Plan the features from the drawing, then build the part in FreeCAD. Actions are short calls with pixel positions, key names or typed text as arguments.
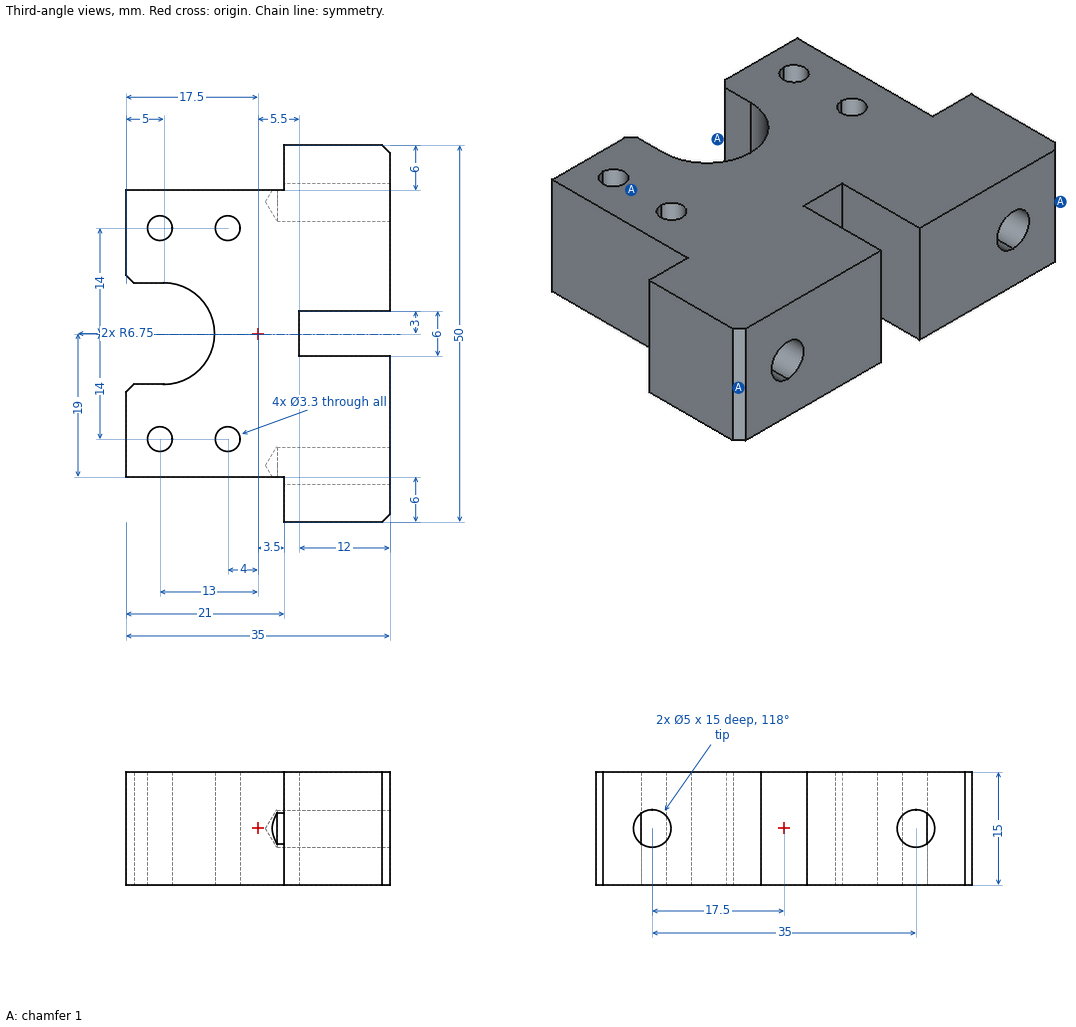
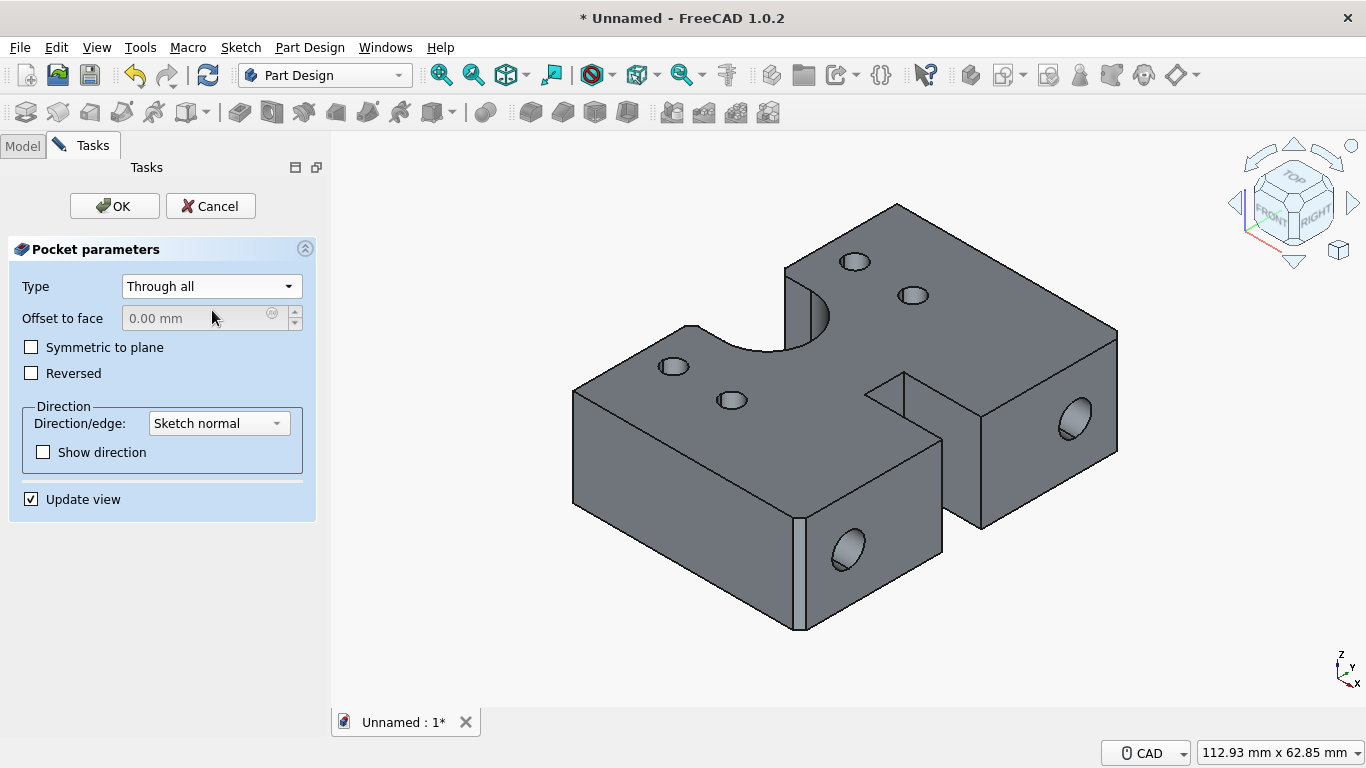
click(115, 206)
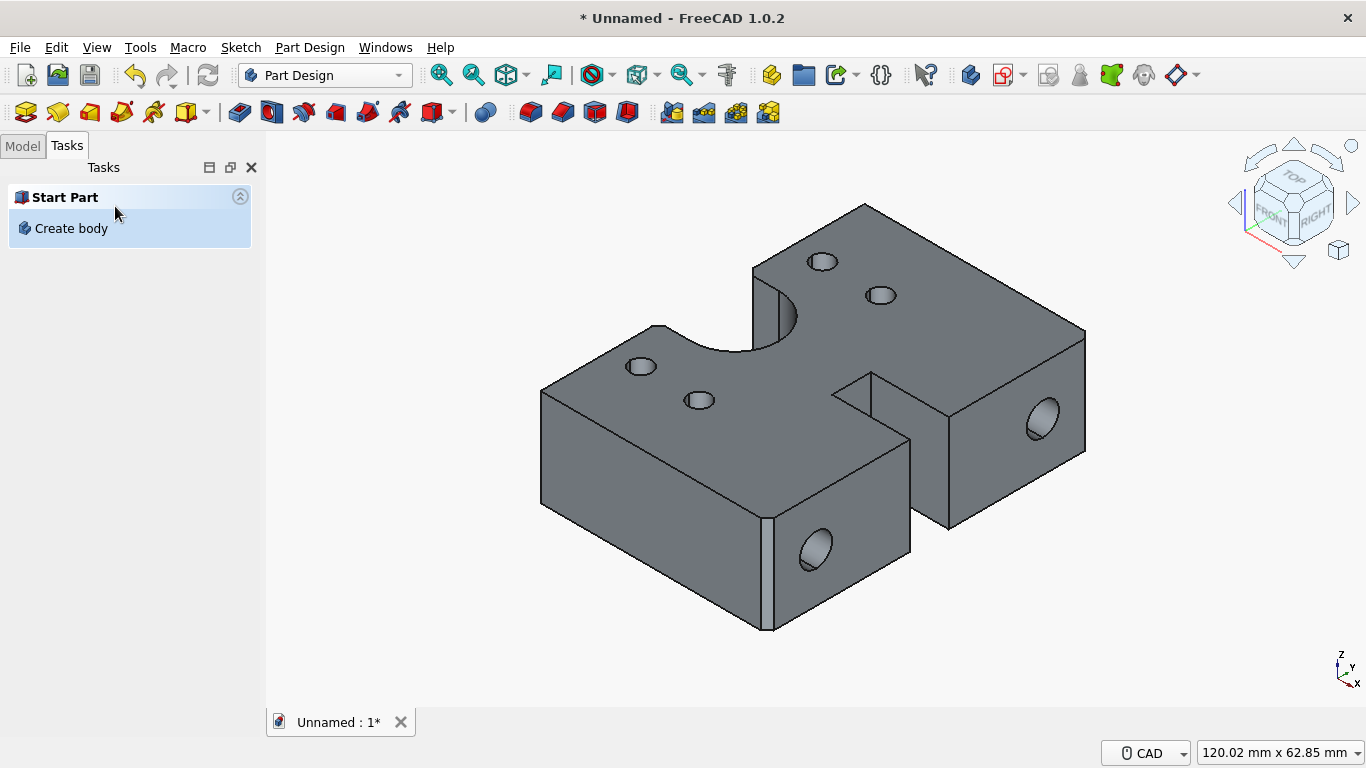
click(973, 346)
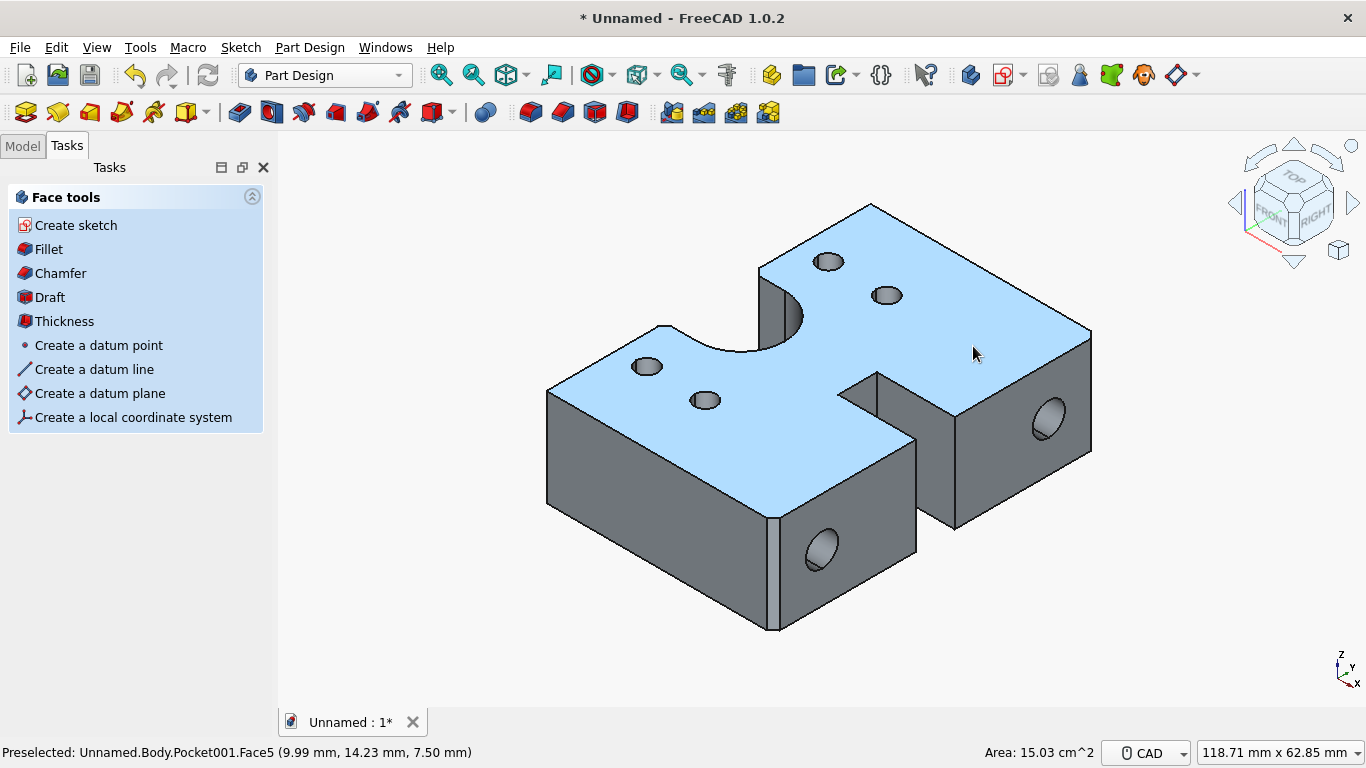
click(1004, 76)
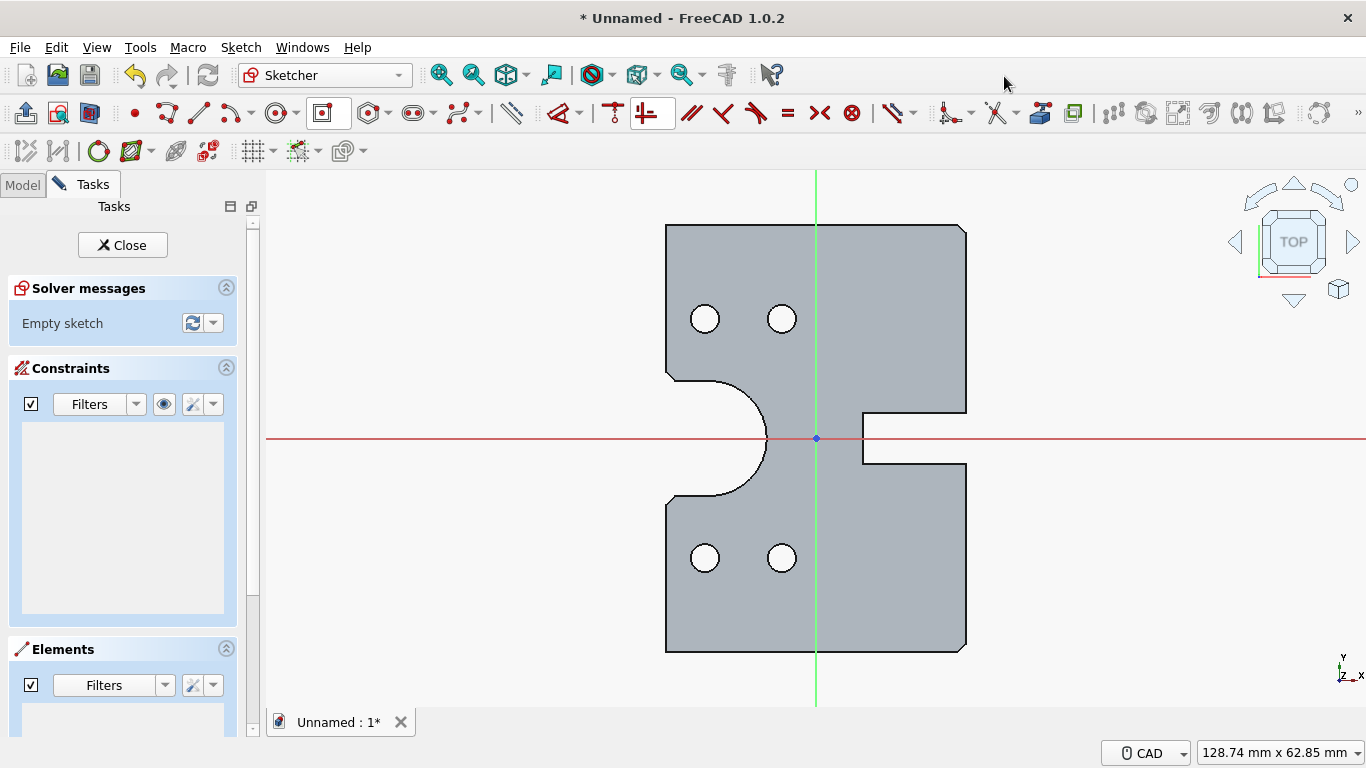
click(346, 114)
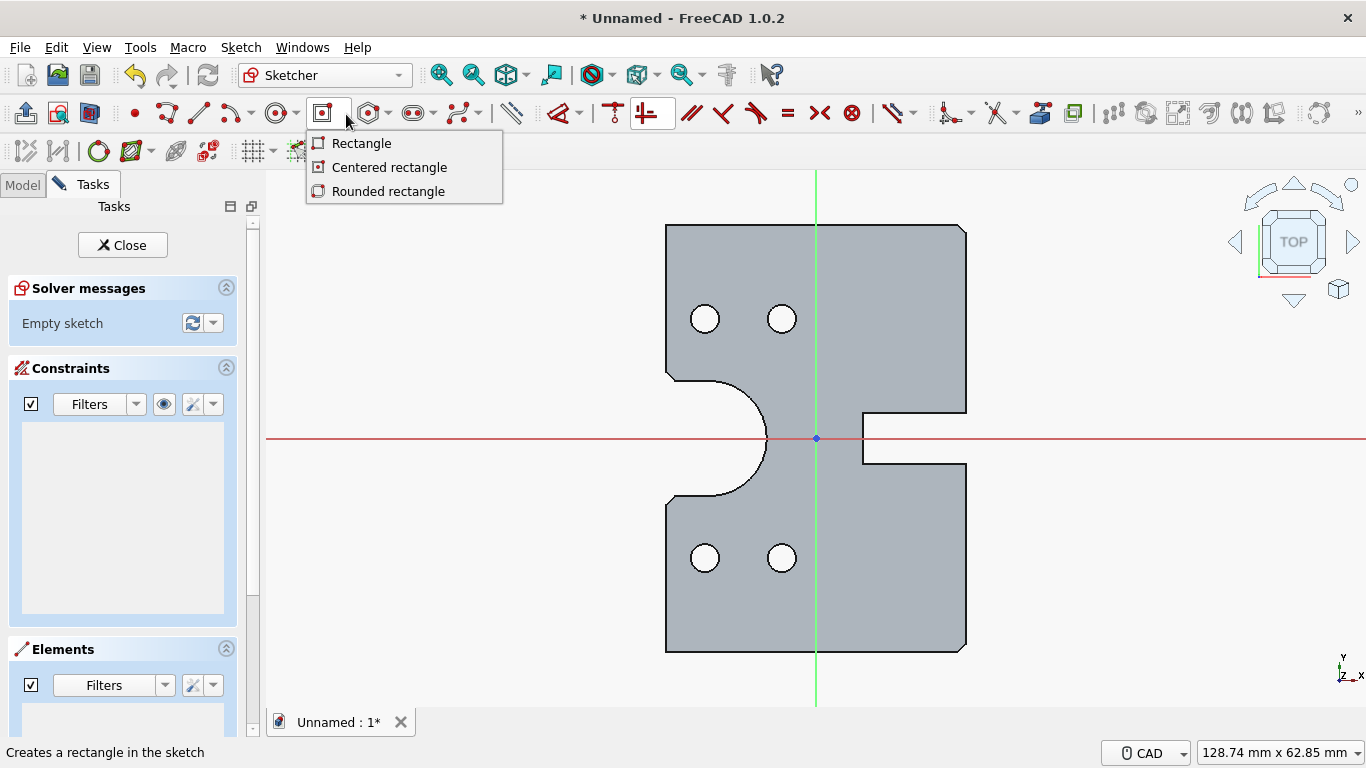
click(404, 143)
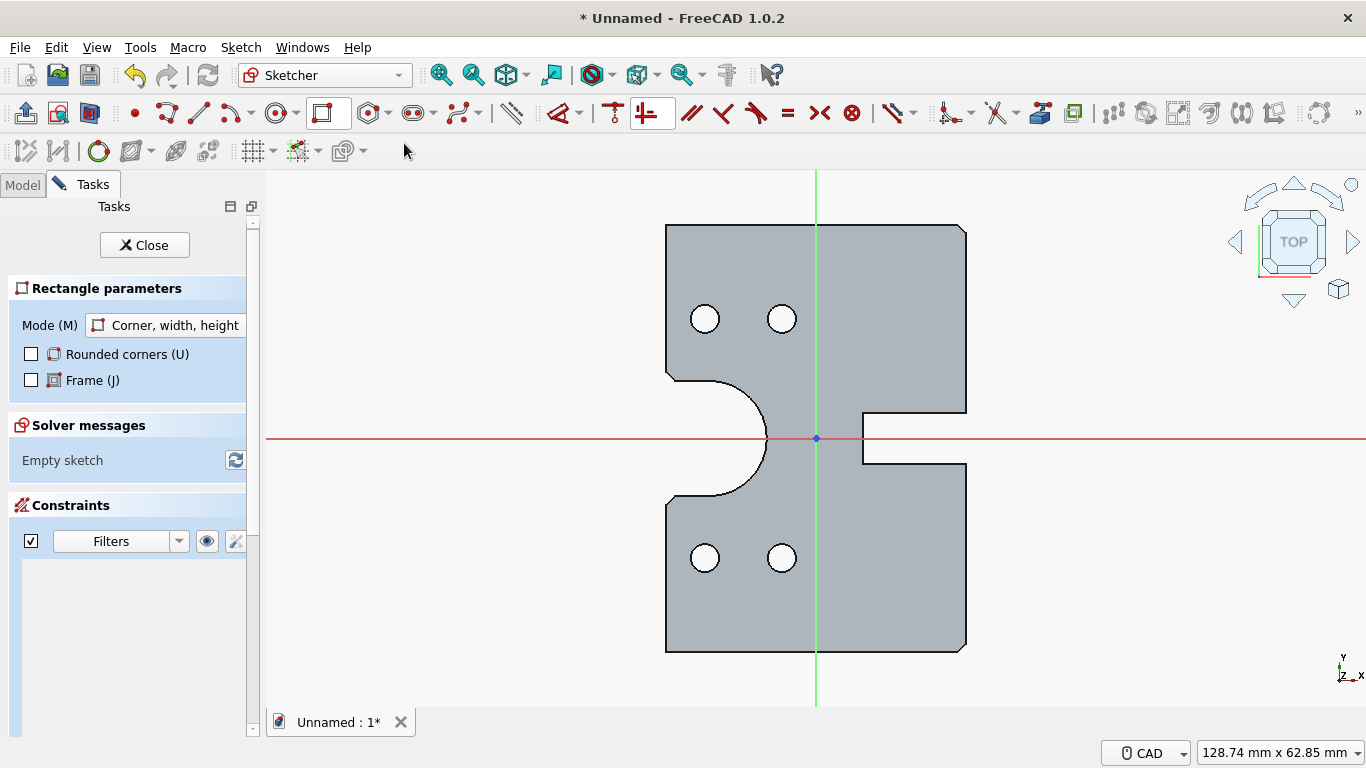
click(666, 601)
move(846, 652)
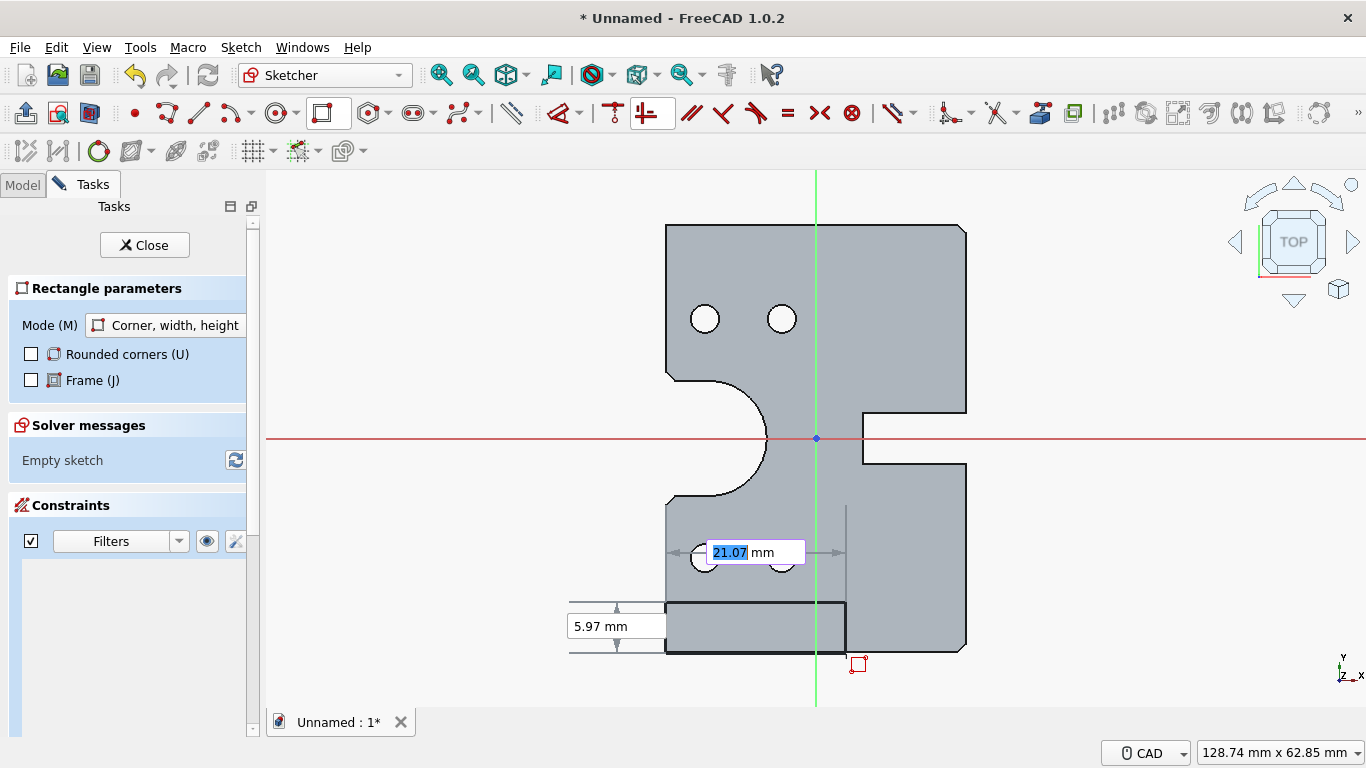
text(21)
key(Tab)
text(6)
key(Return)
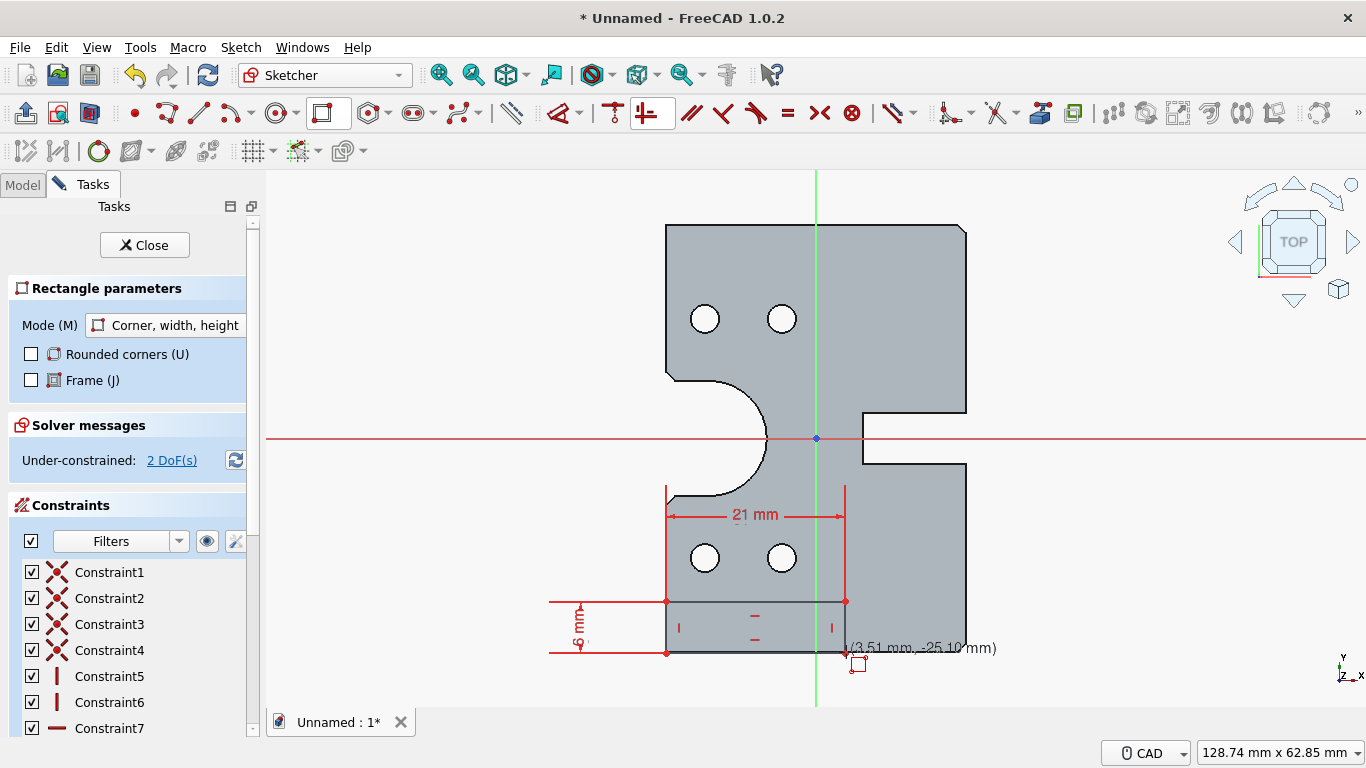
click(666, 225)
move(846, 276)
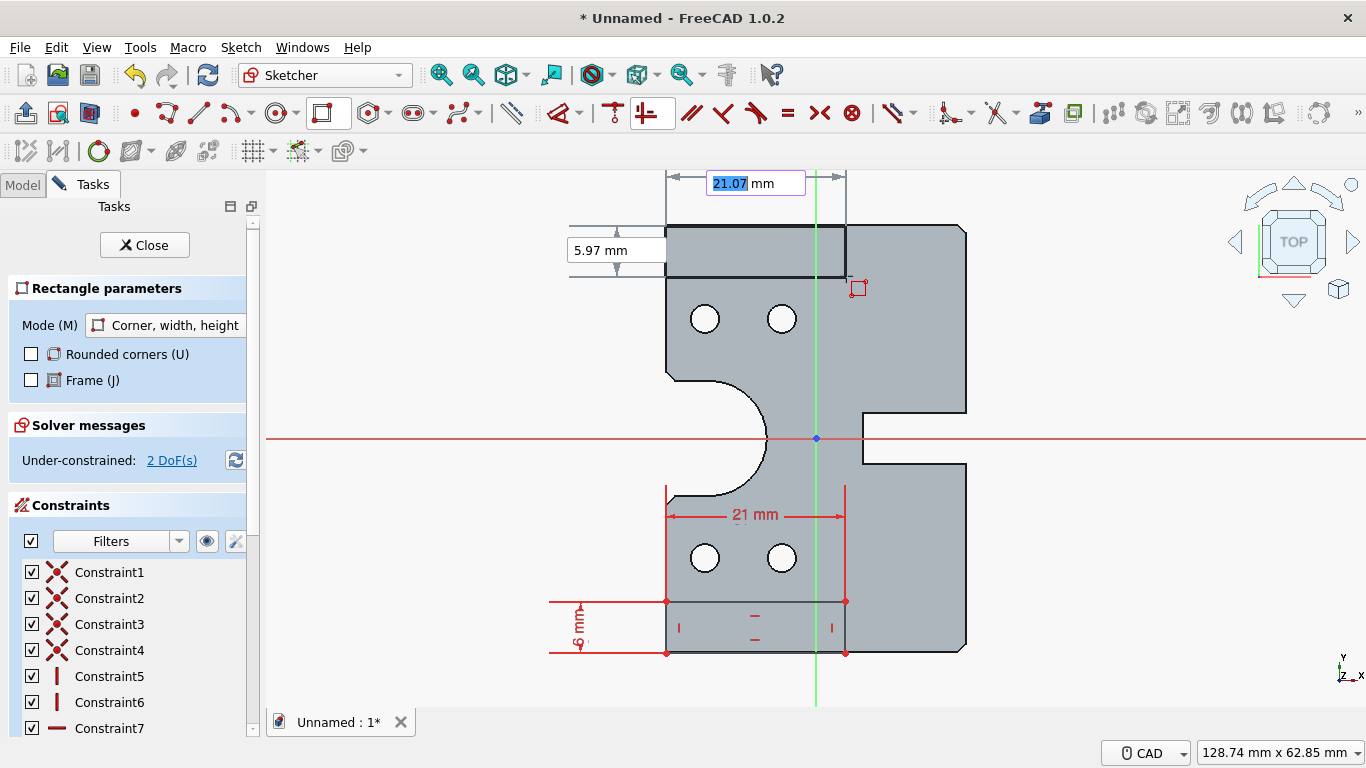
text(21)
key(Tab)
text(6)
key(Return)
key(Escape)